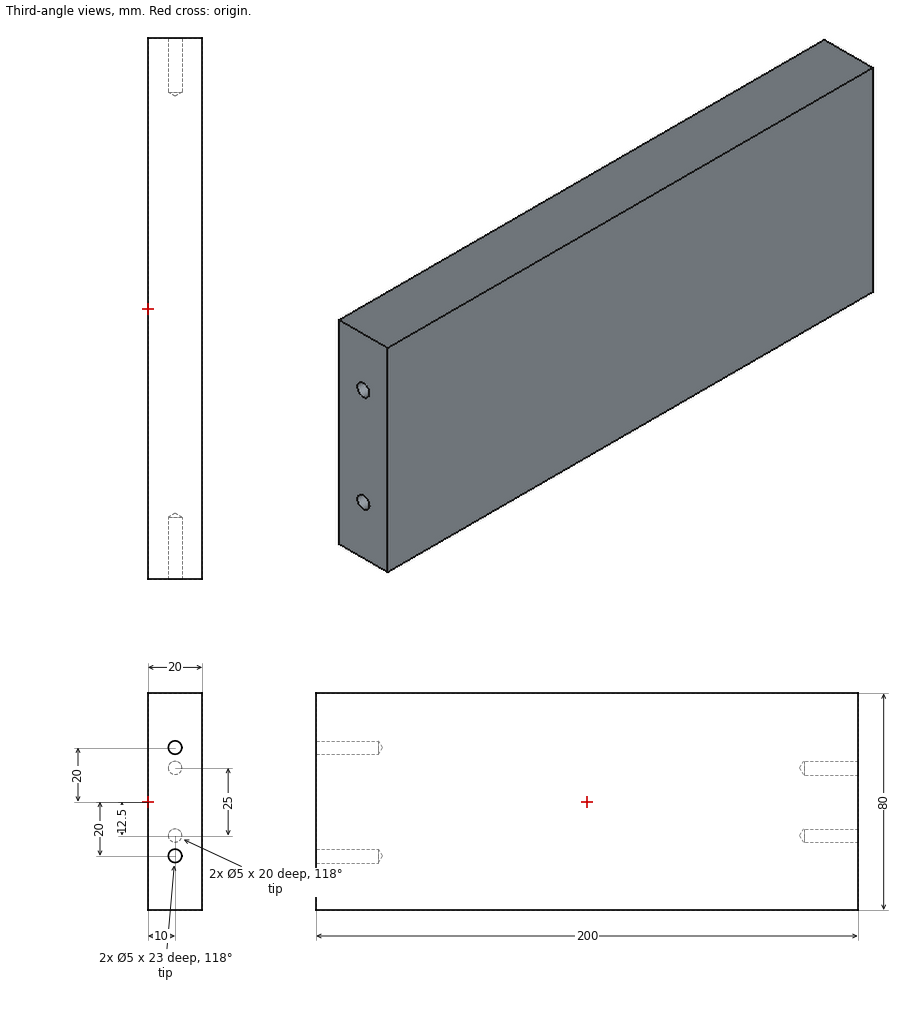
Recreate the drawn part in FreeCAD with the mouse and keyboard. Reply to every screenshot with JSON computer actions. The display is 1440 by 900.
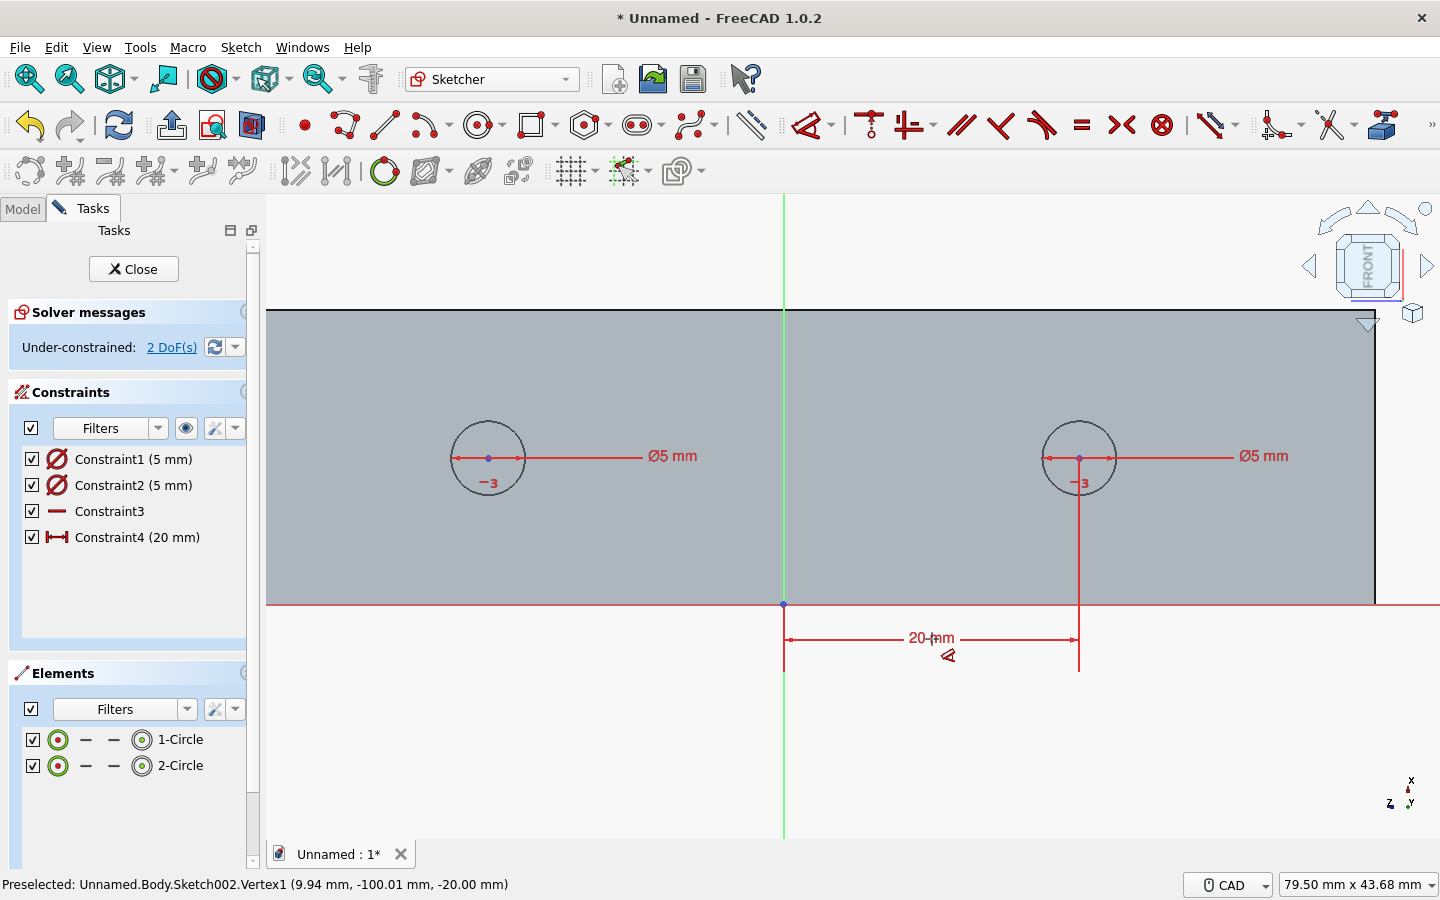
{"action": "left_click", "coordinate": [1079, 458]}
{"action": "left_click", "coordinate": [1113, 532]}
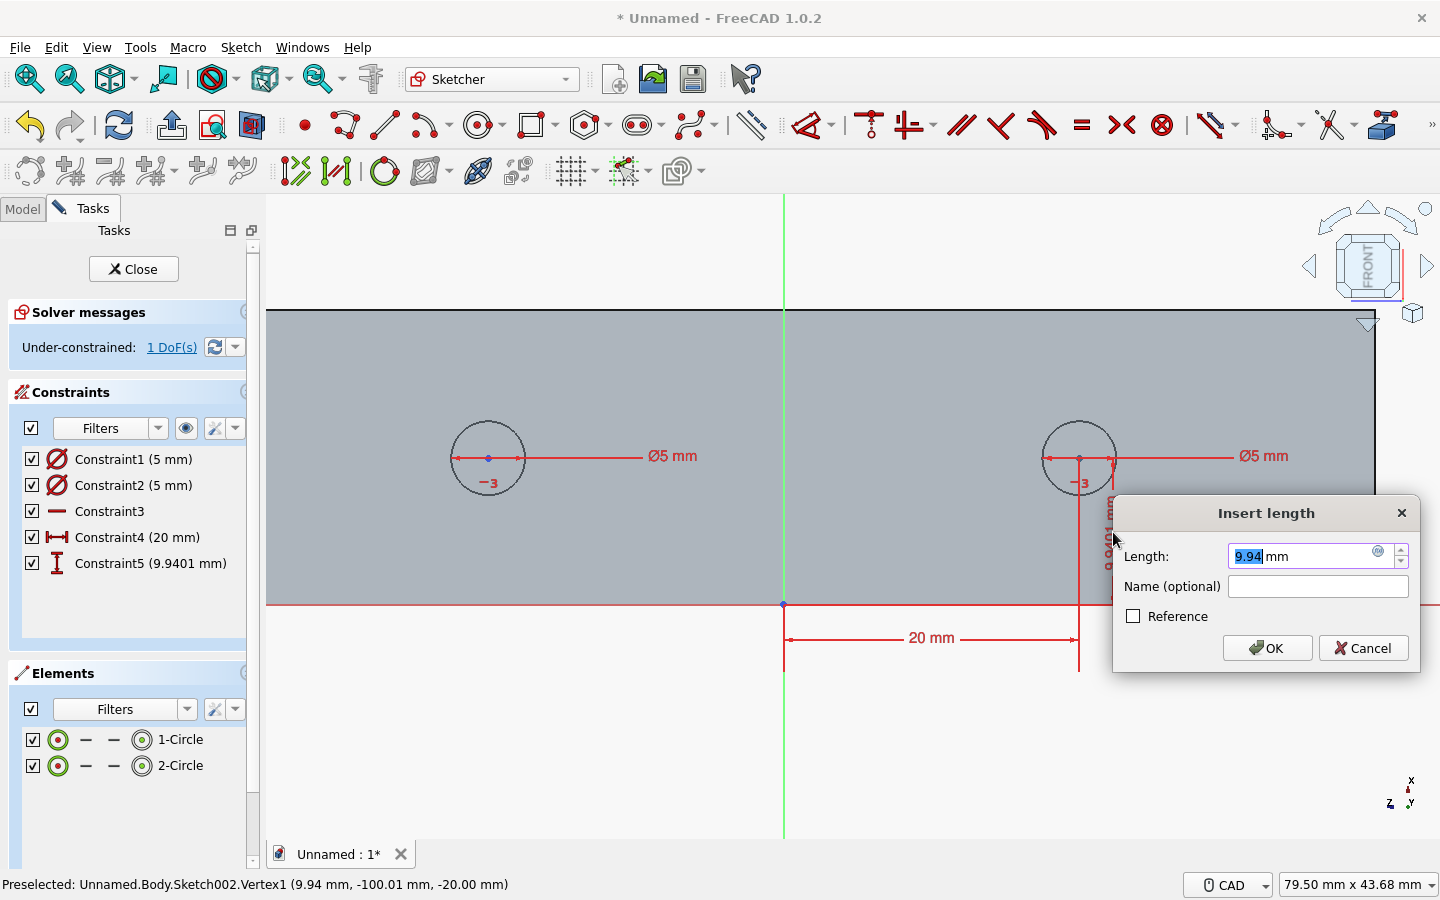
{"action": "type", "text": "10"}
{"action": "key", "text": "Return"}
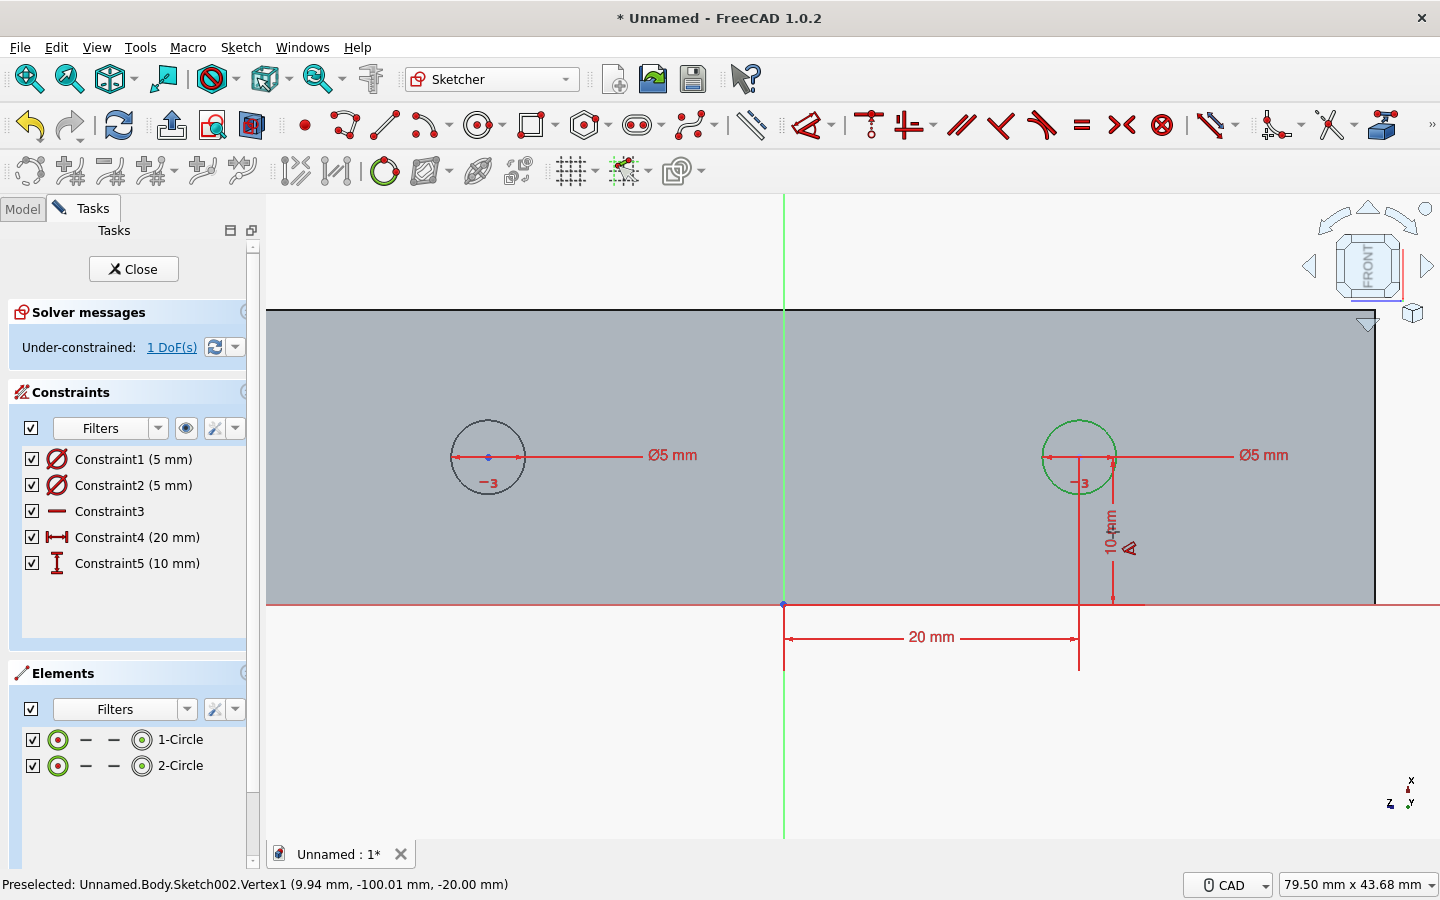
{"action": "left_click", "coordinate": [488, 457]}
{"action": "left_click", "coordinate": [636, 639]}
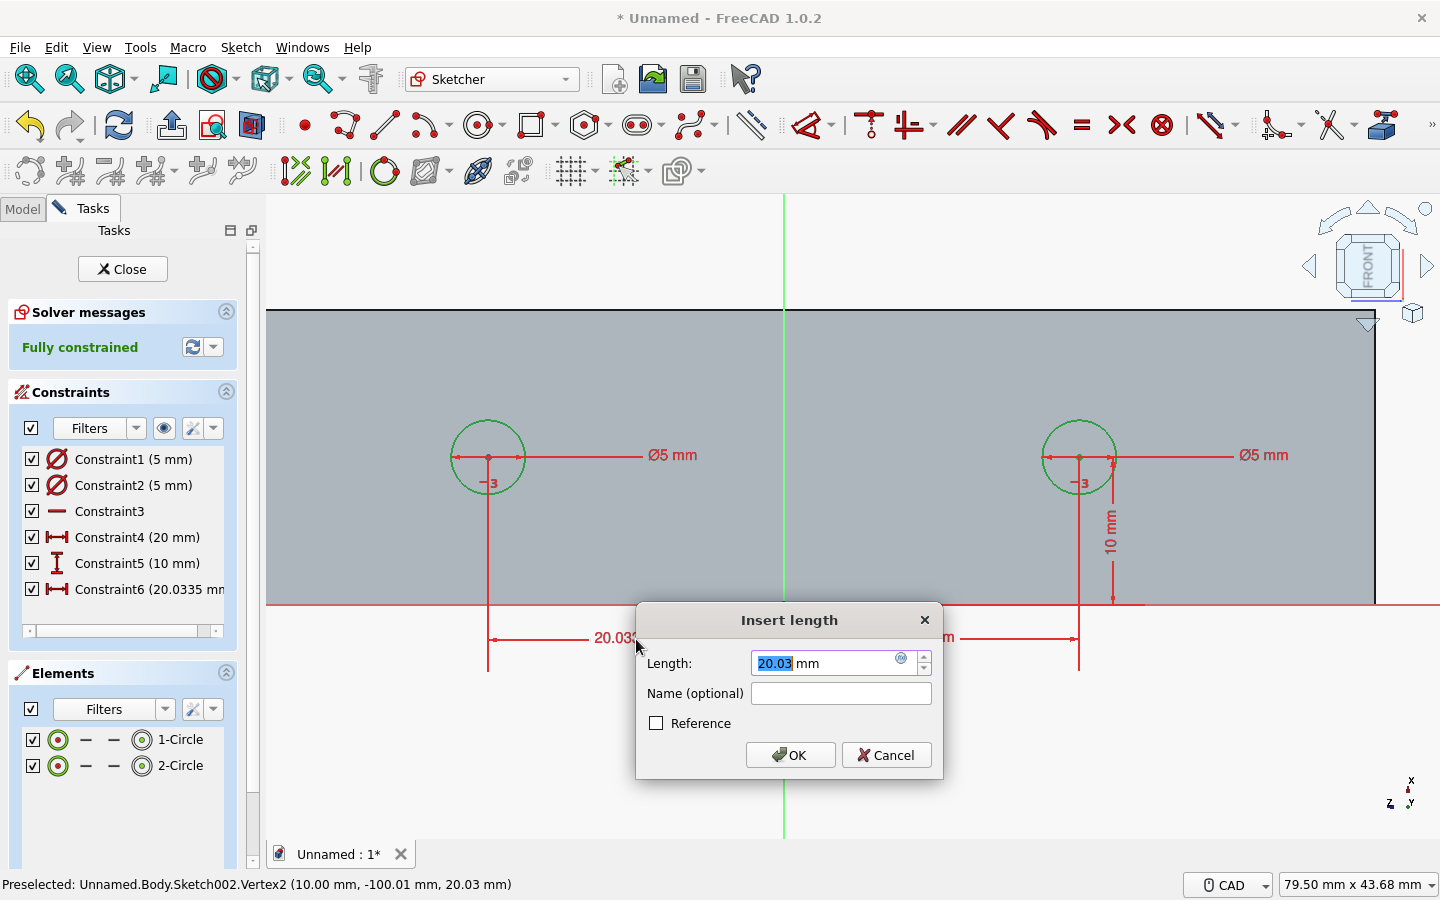
{"action": "type", "text": "20"}
{"action": "key", "text": "Return"}
{"action": "key", "text": "Escape"}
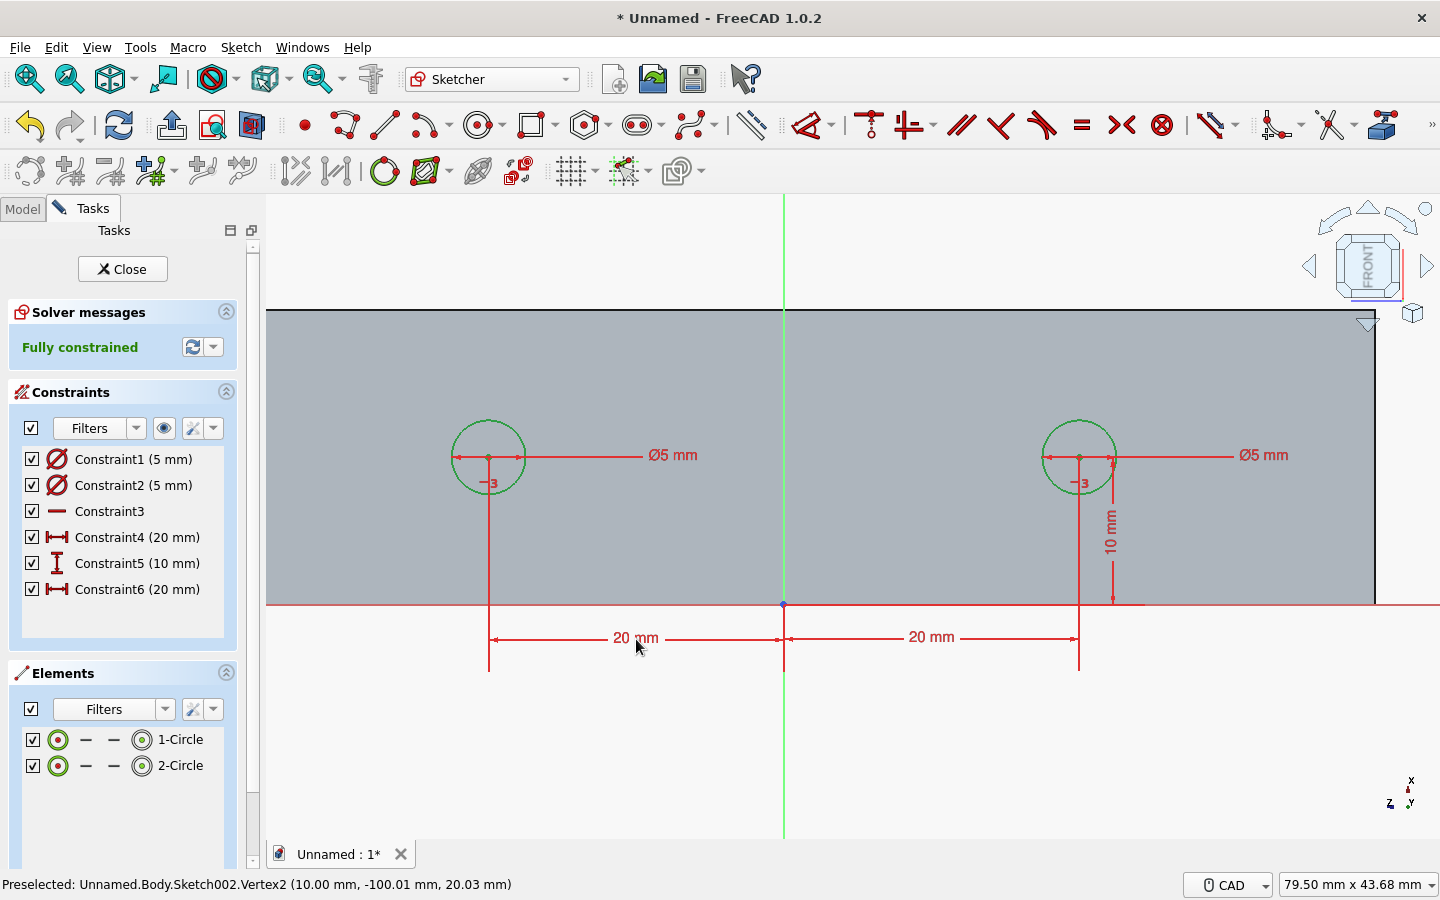
{"action": "left_click", "coordinate": [123, 269]}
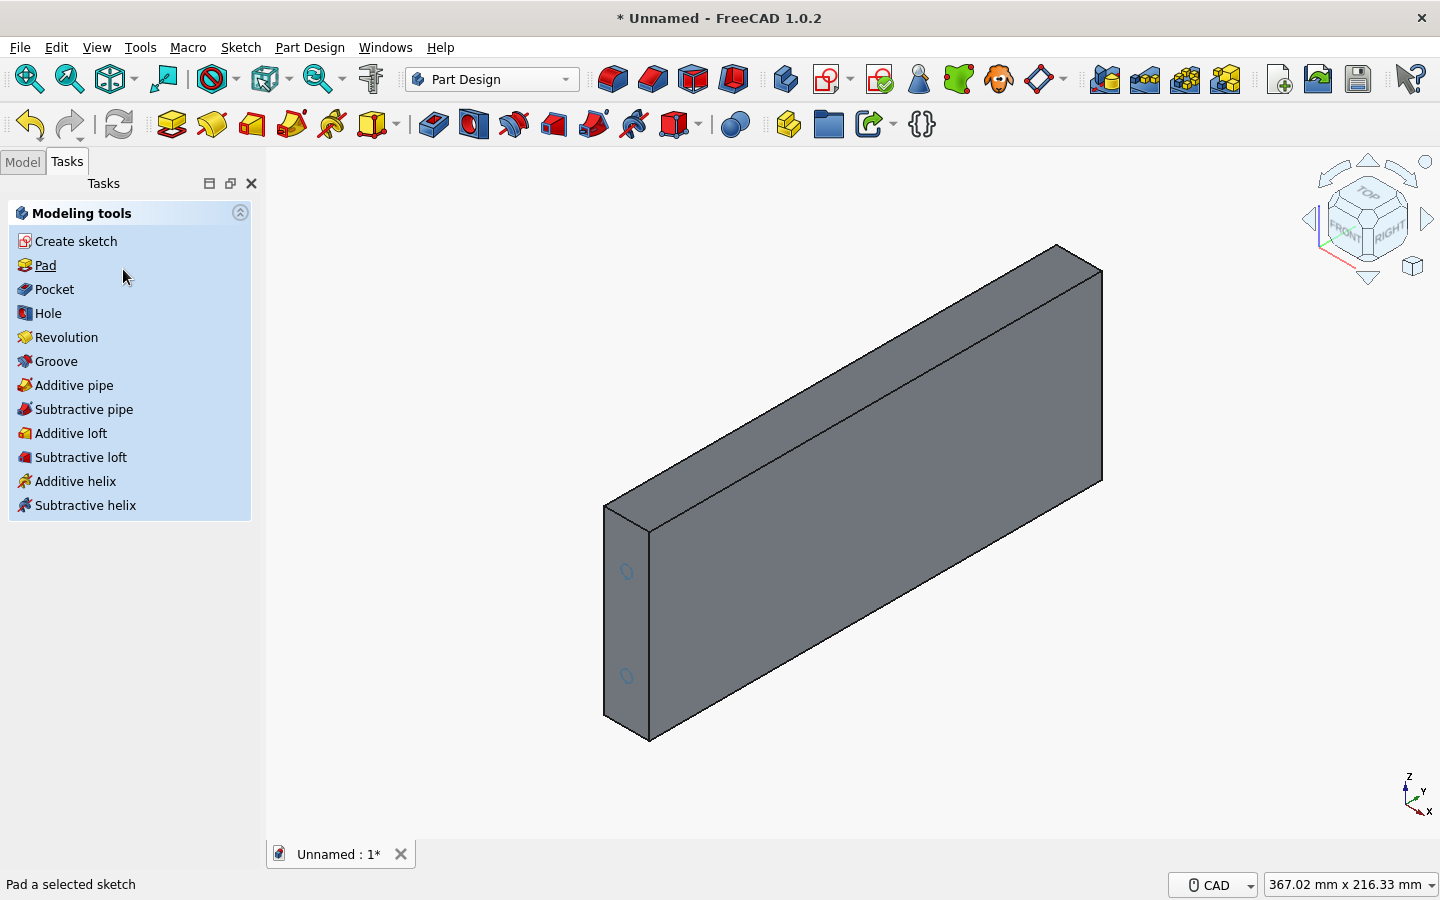
{"action": "left_click", "coordinate": [474, 124]}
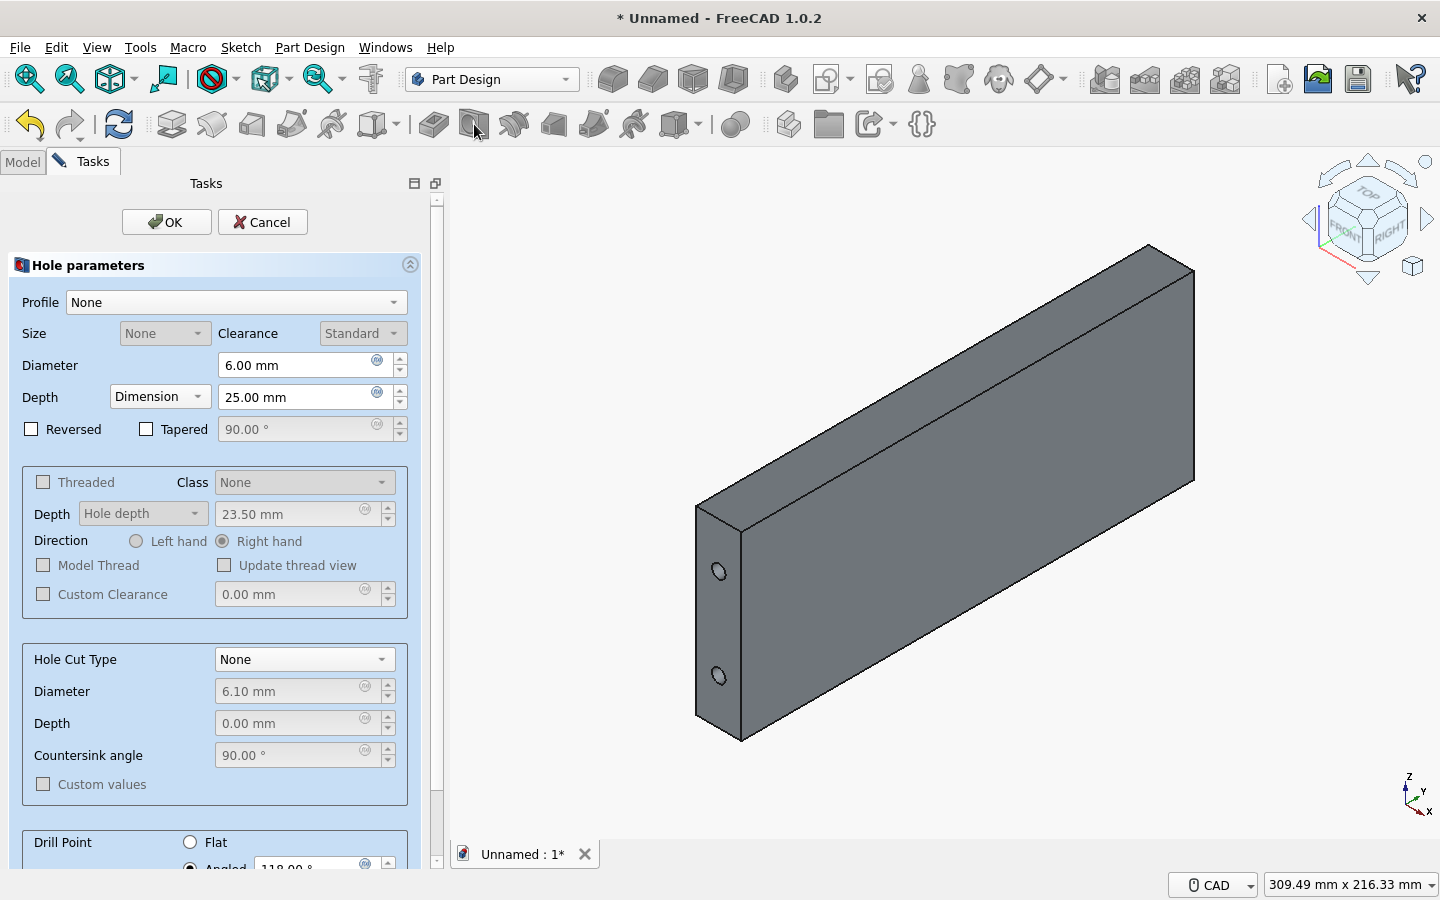
{"action": "triple_click", "coordinate": [305, 365]}